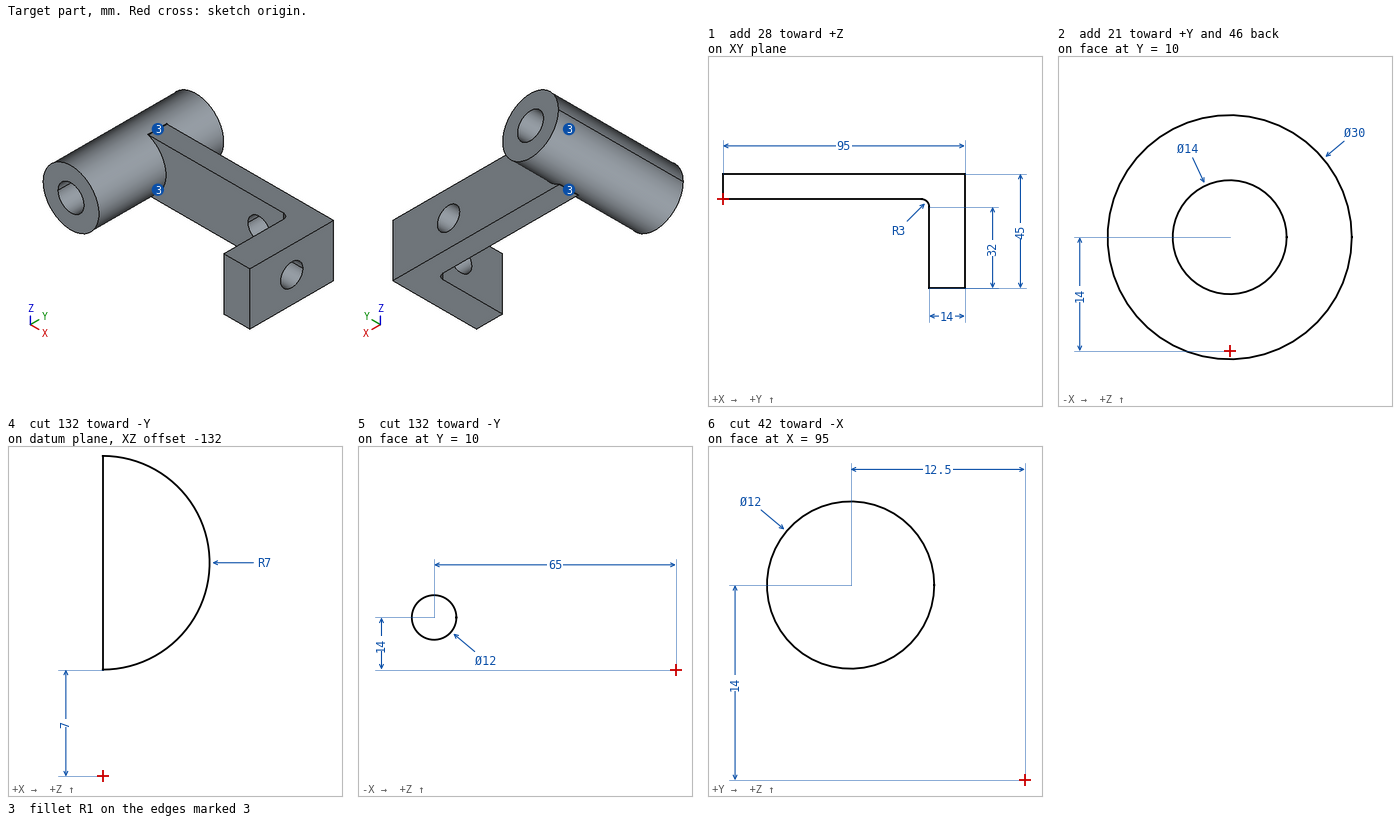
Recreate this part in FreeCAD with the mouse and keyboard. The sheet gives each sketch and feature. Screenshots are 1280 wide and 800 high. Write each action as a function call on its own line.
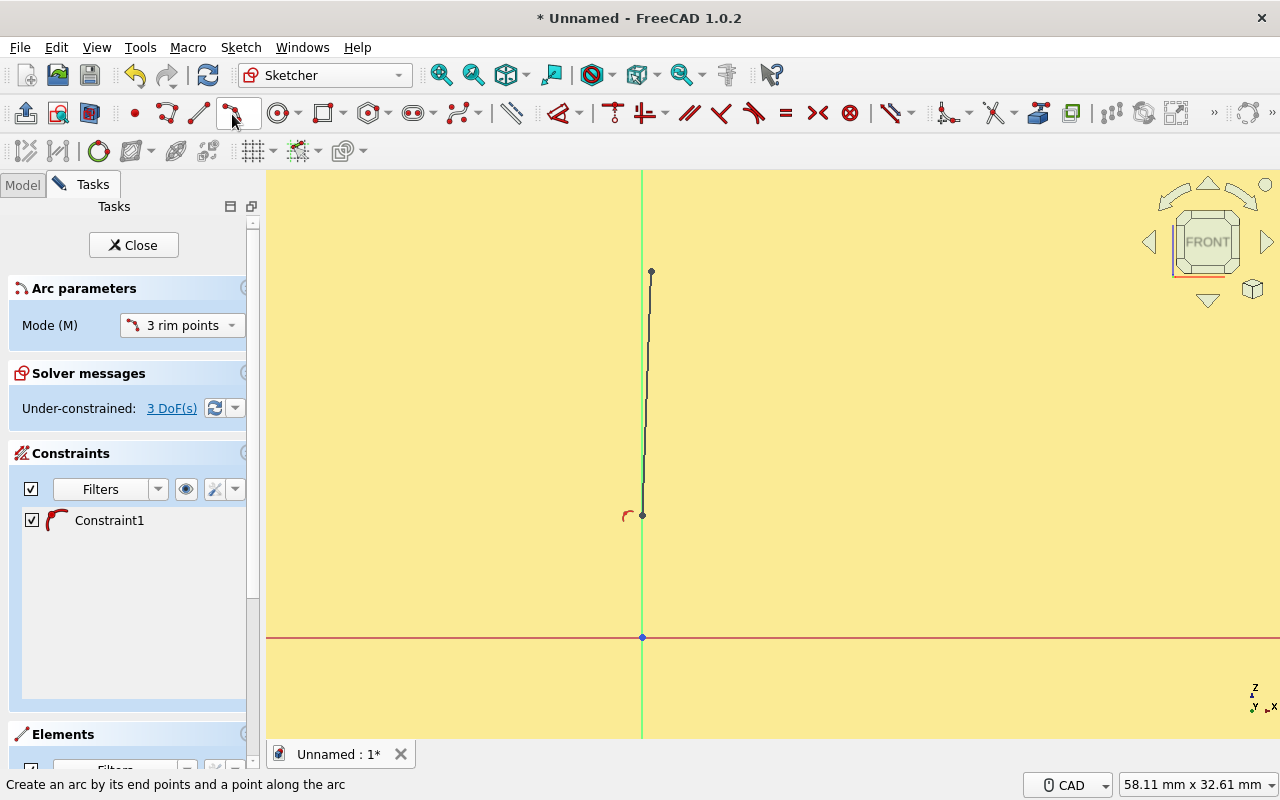
click(651, 272)
click(642, 516)
click(764, 393)
key(Escape)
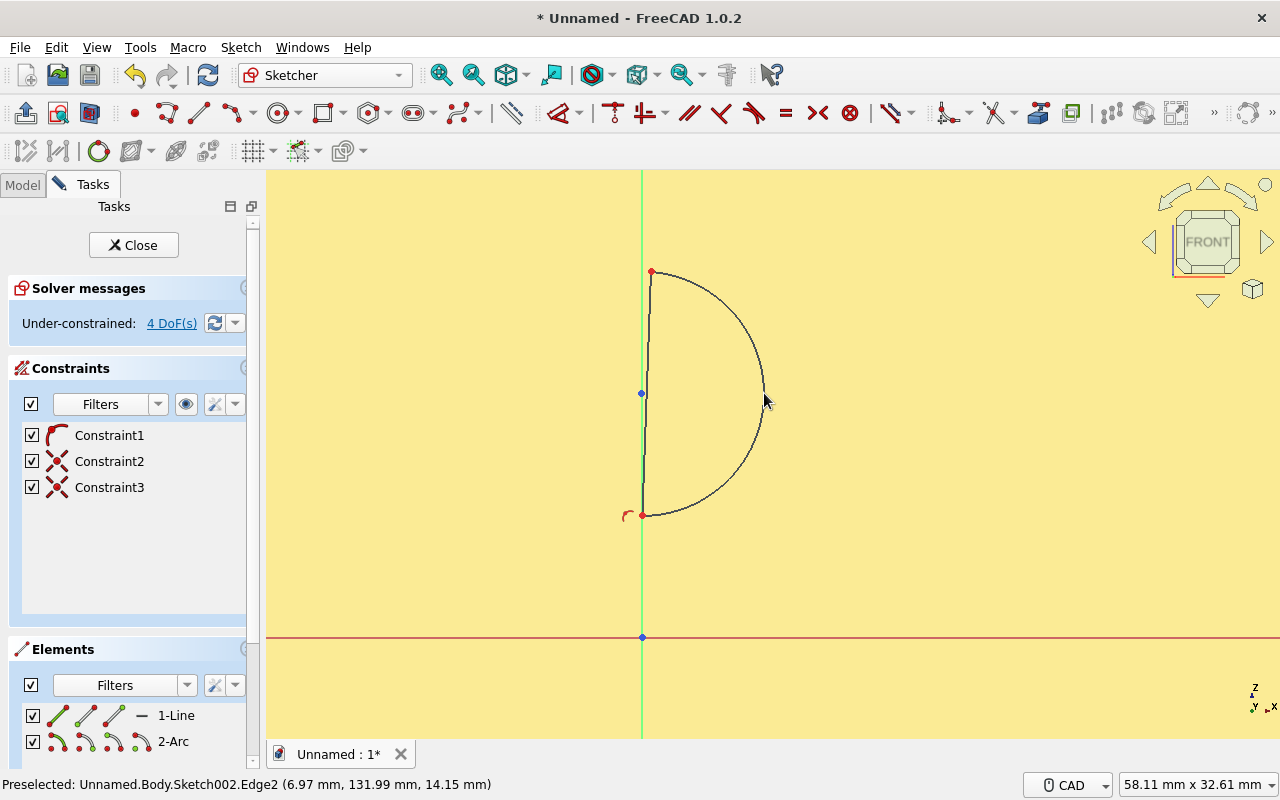
click(645, 443)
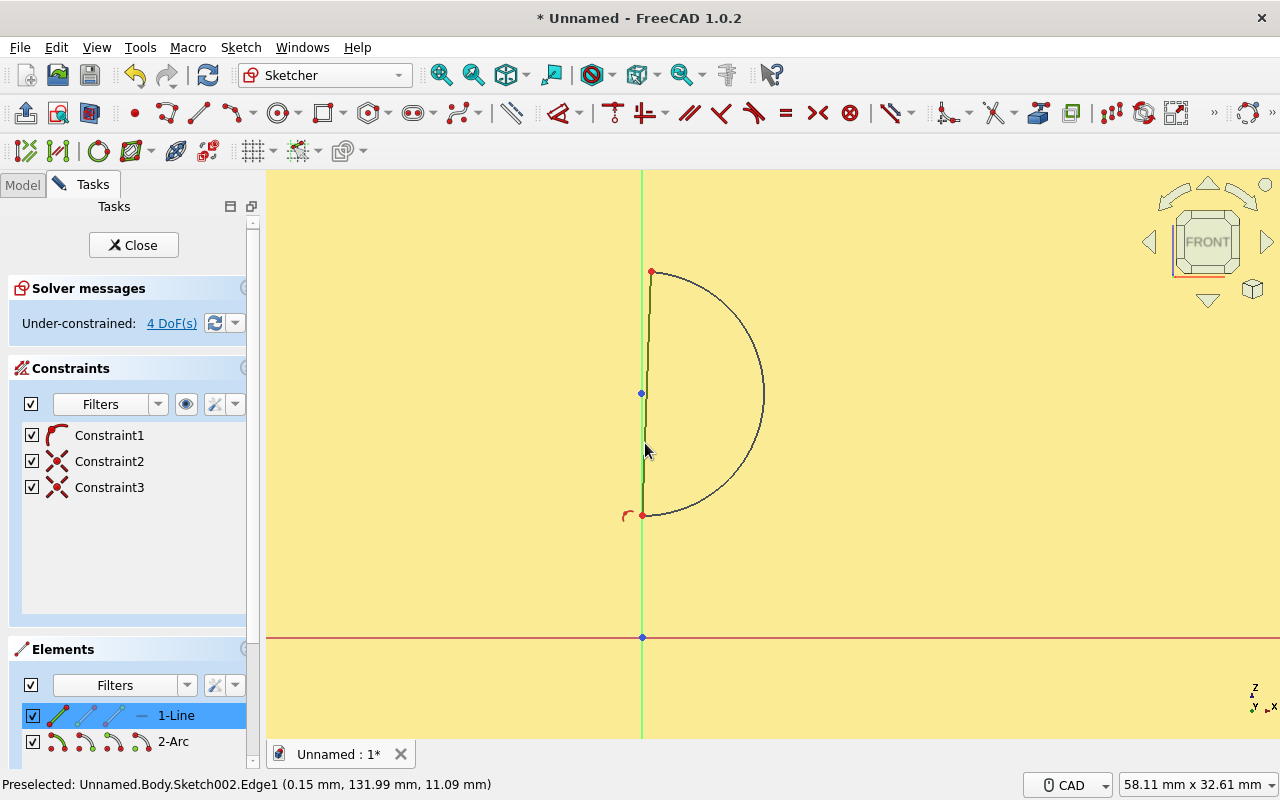
click(668, 114)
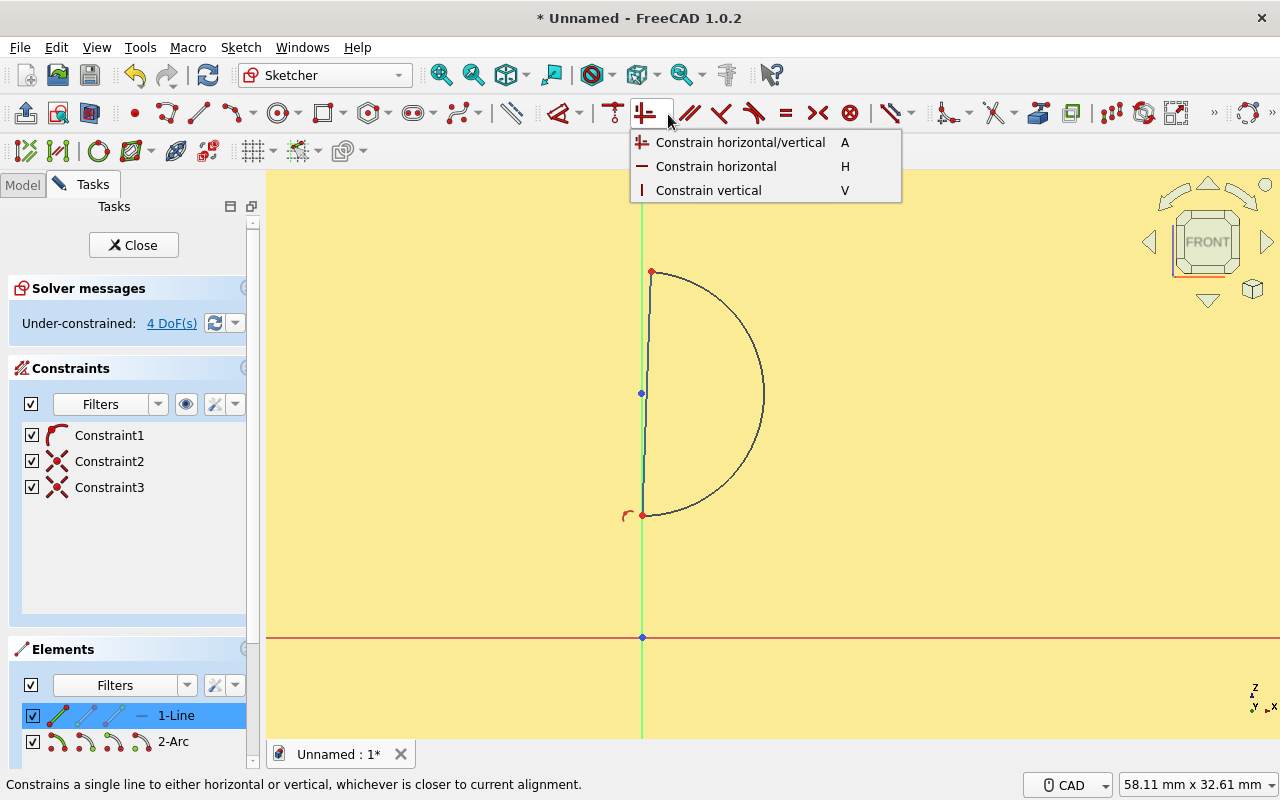
click(766, 190)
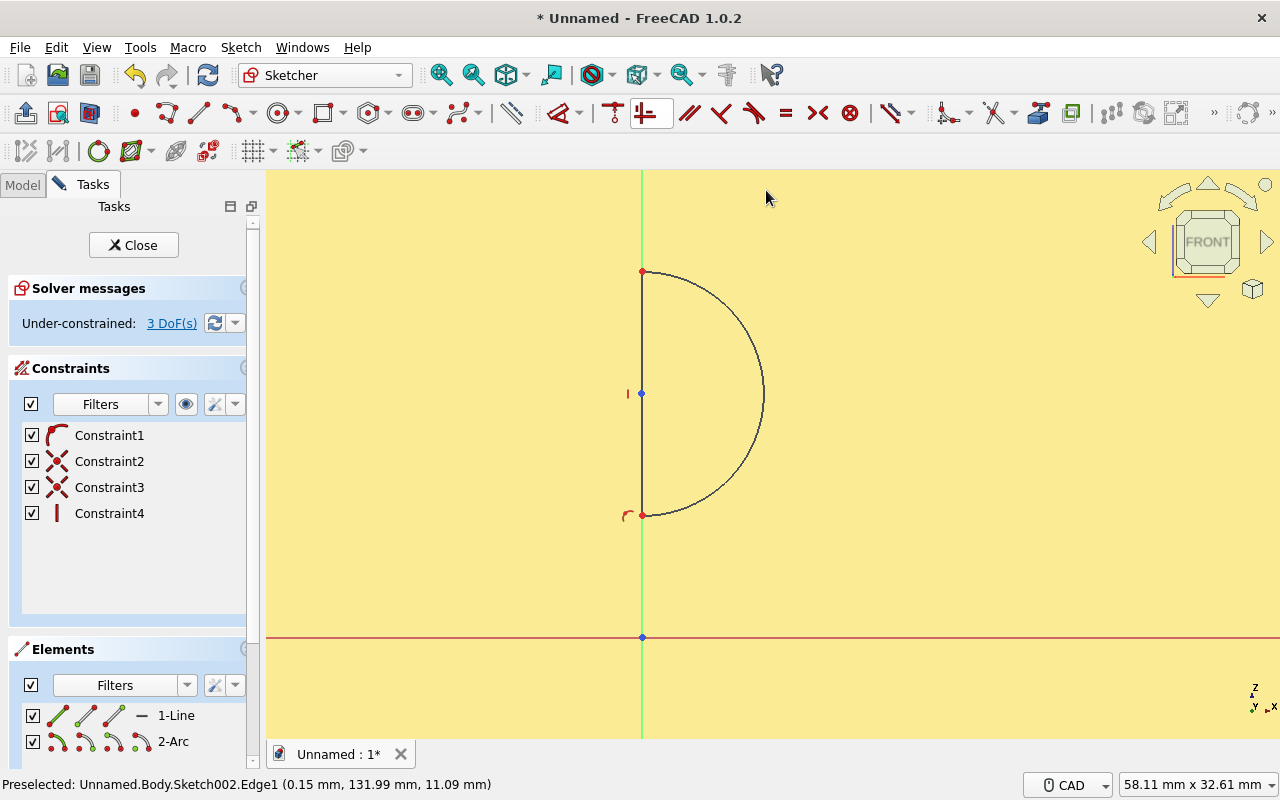
click(642, 394)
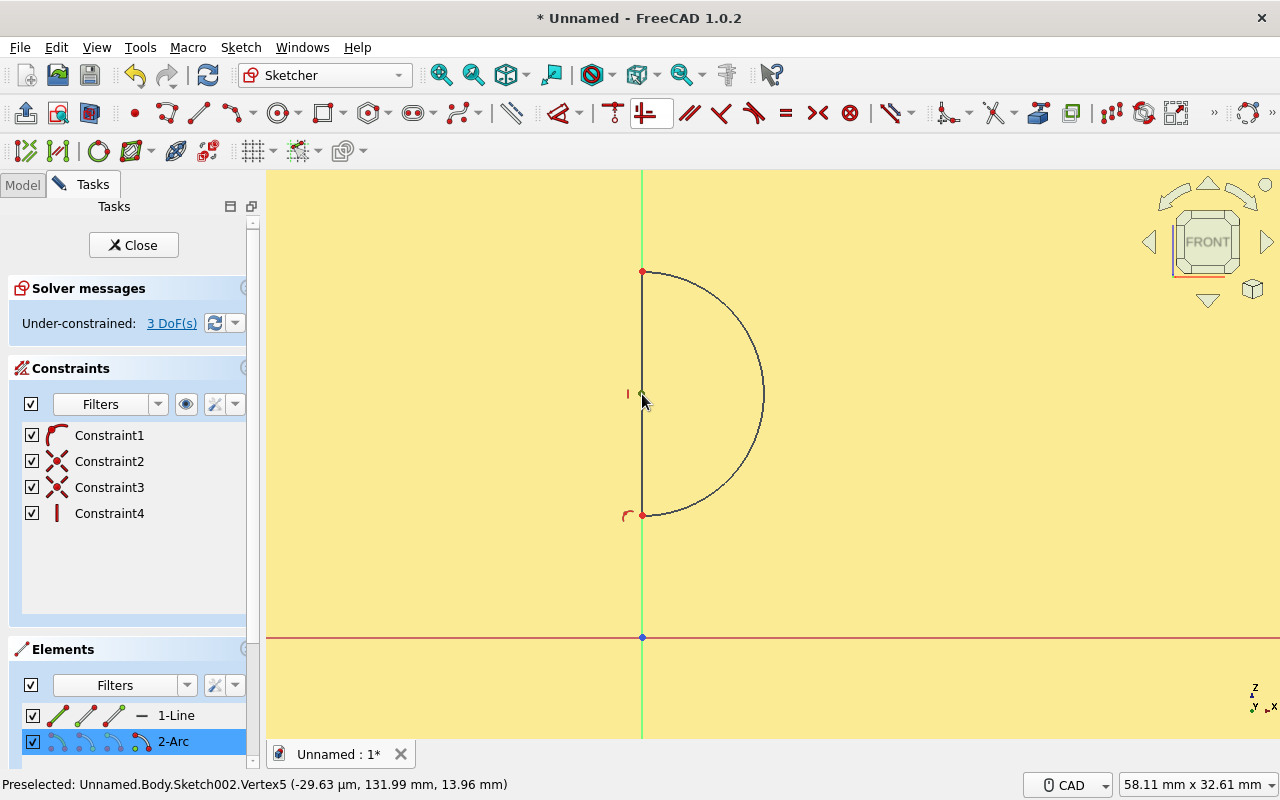
click(642, 674)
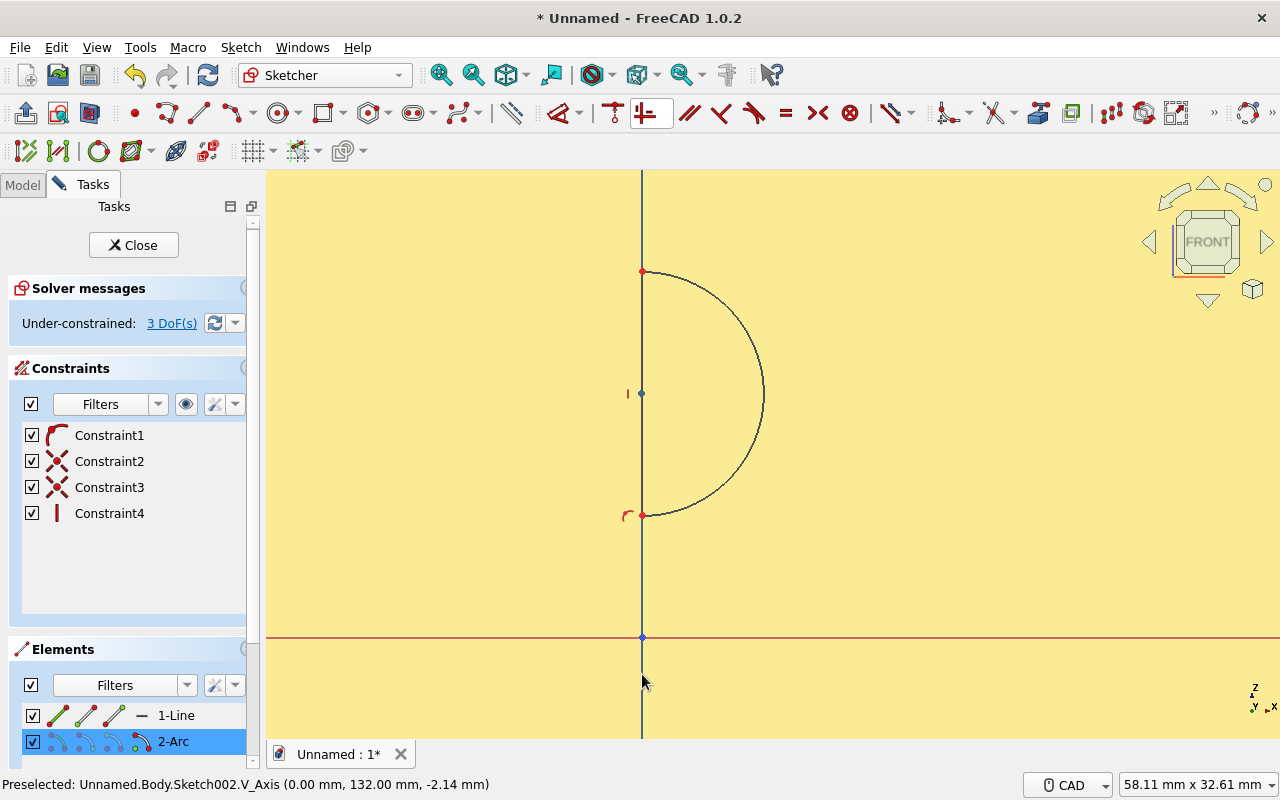
click(614, 114)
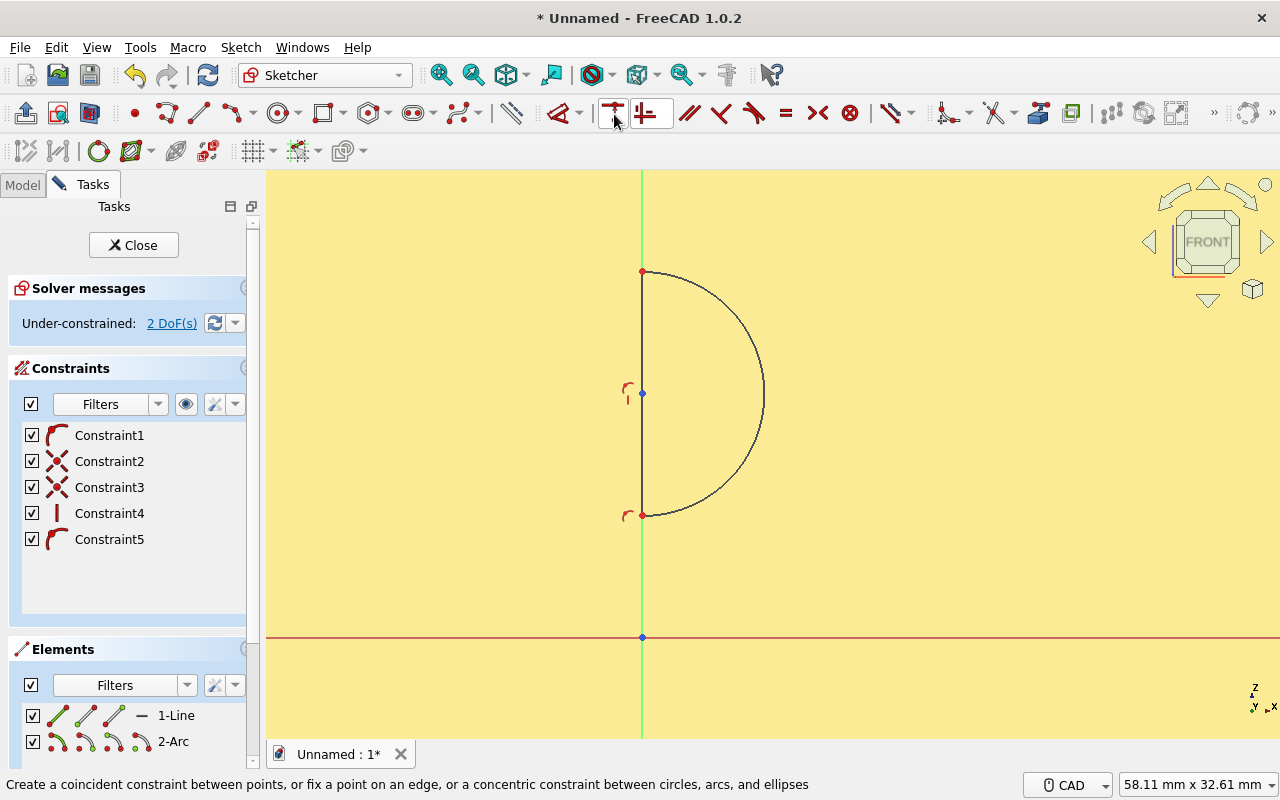
click(558, 114)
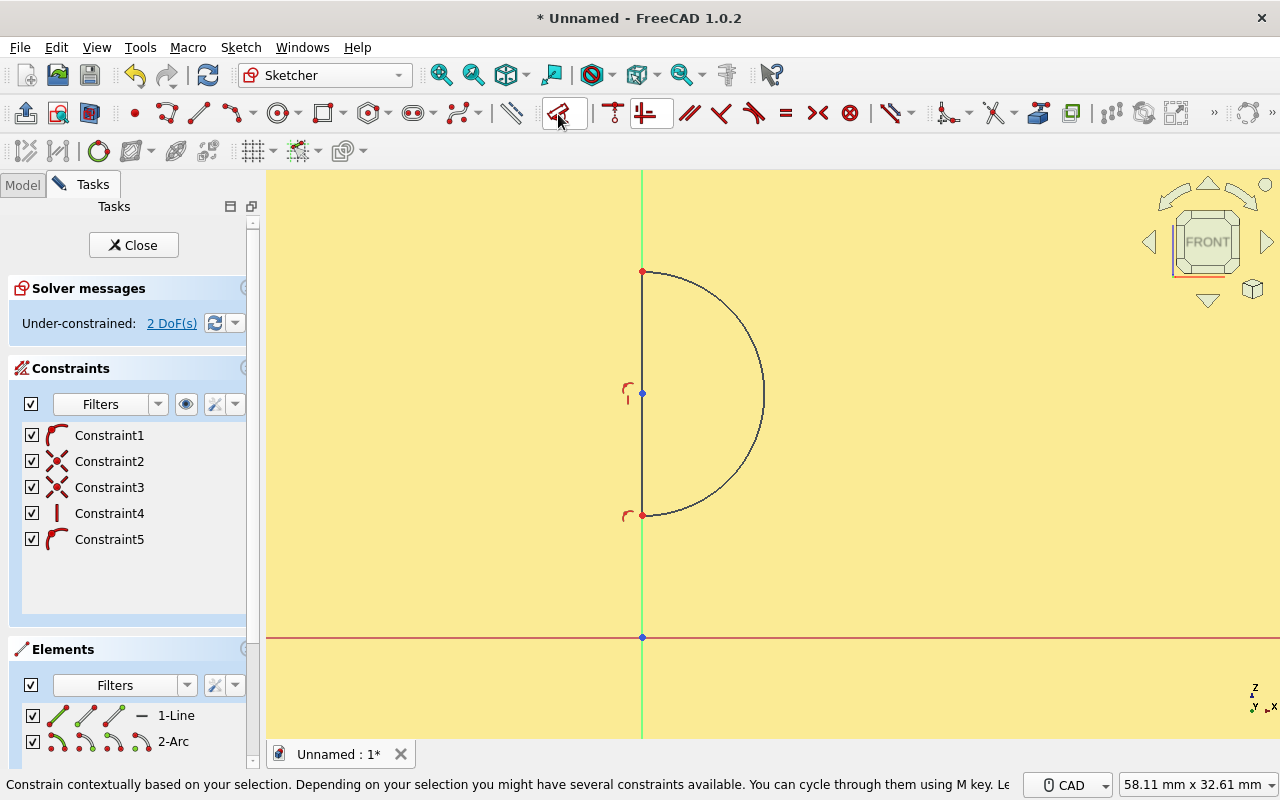
click(741, 466)
click(767, 485)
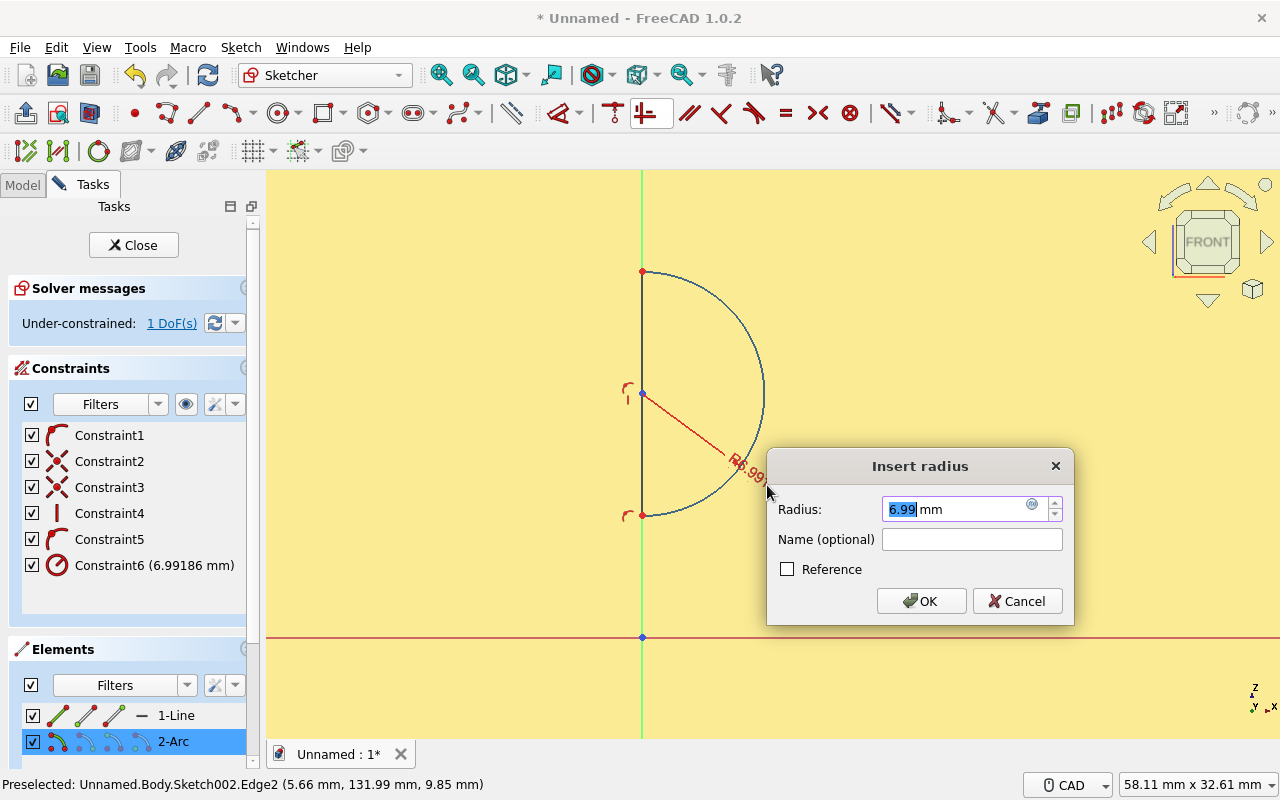
text(7)
key(Return)